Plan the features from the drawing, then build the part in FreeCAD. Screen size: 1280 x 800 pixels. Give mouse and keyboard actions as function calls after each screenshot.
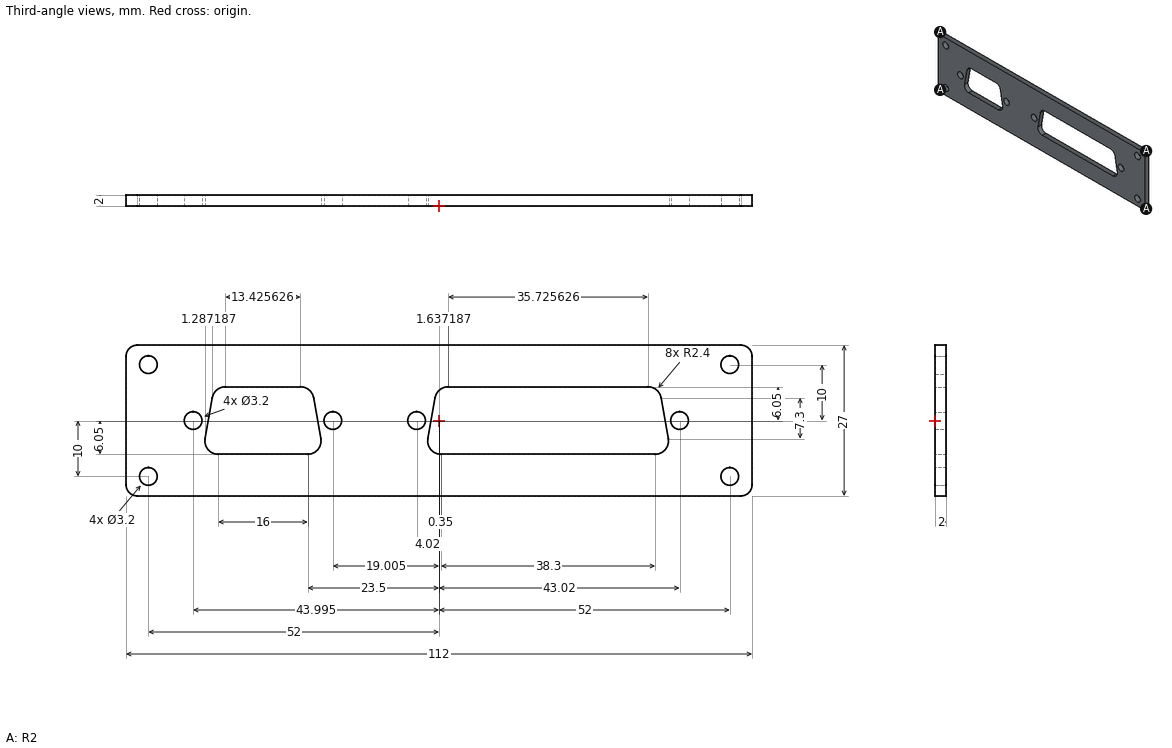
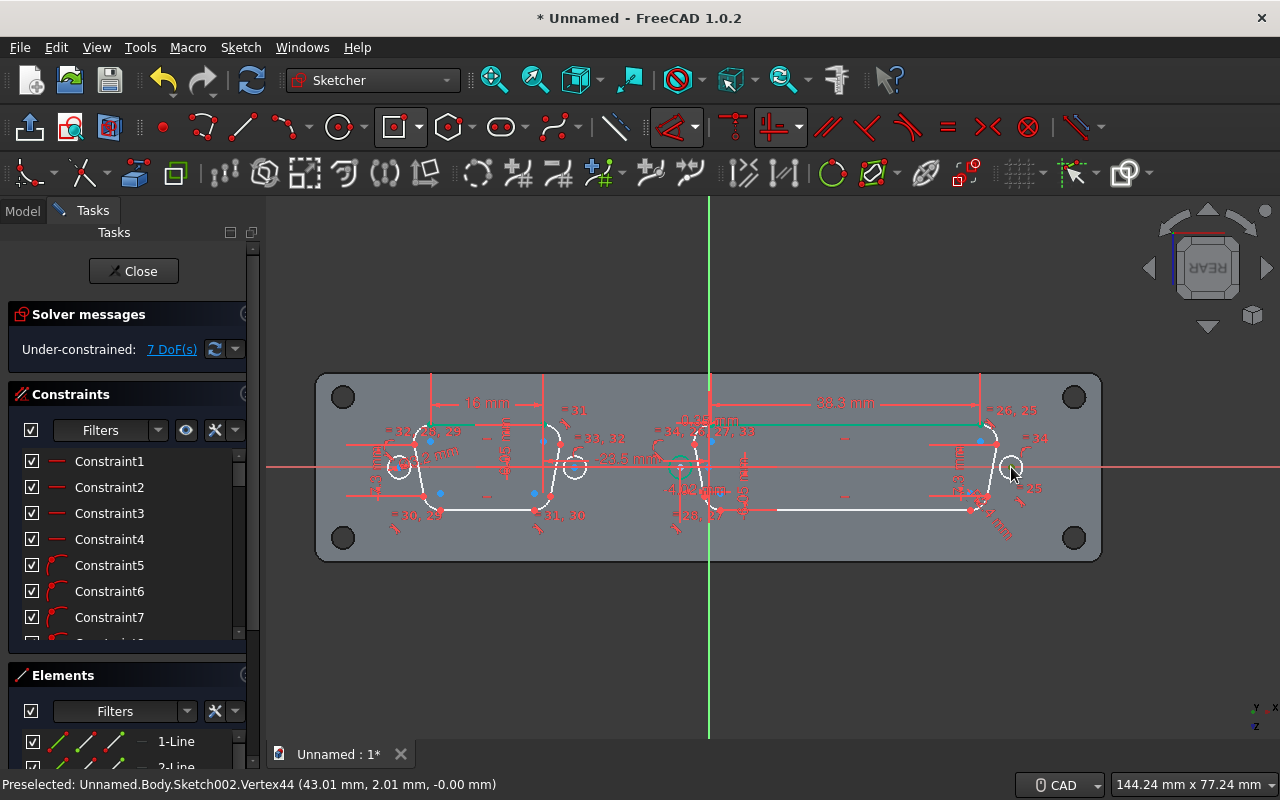
click(698, 128)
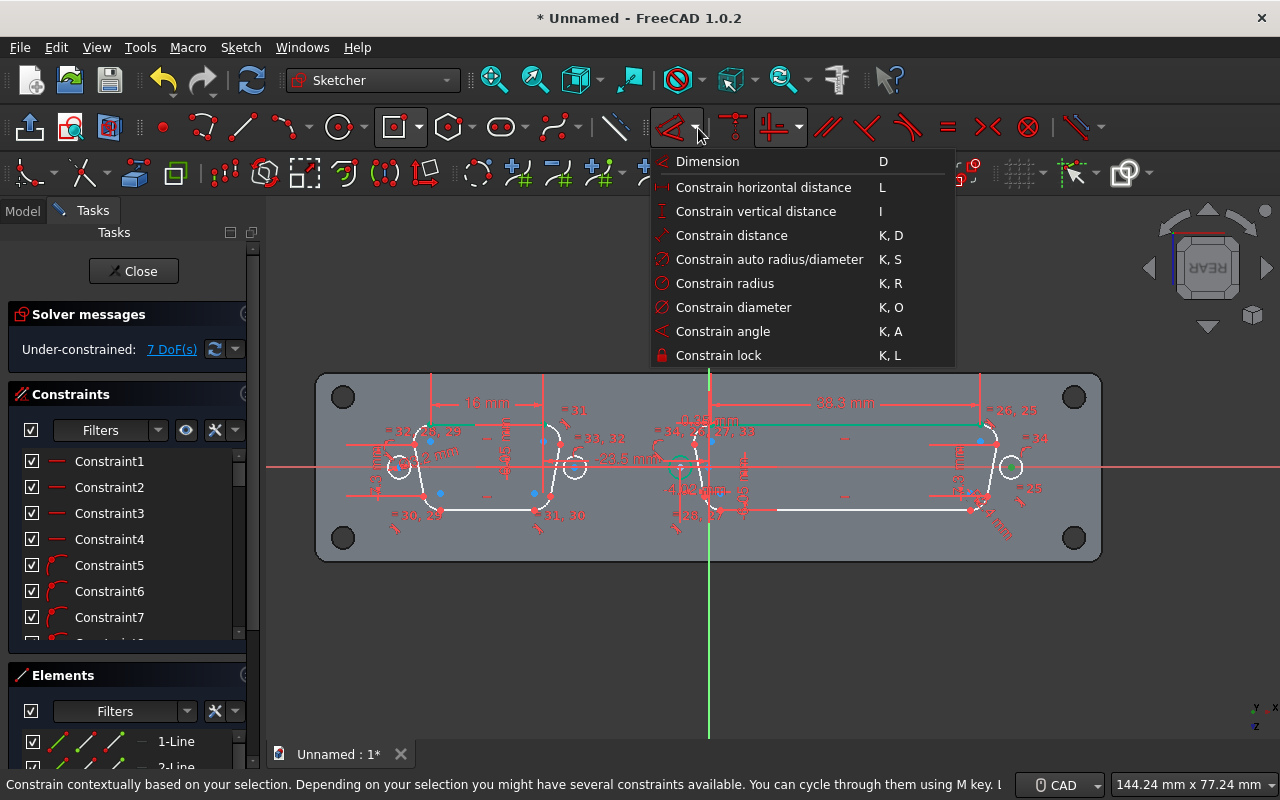
click(803, 187)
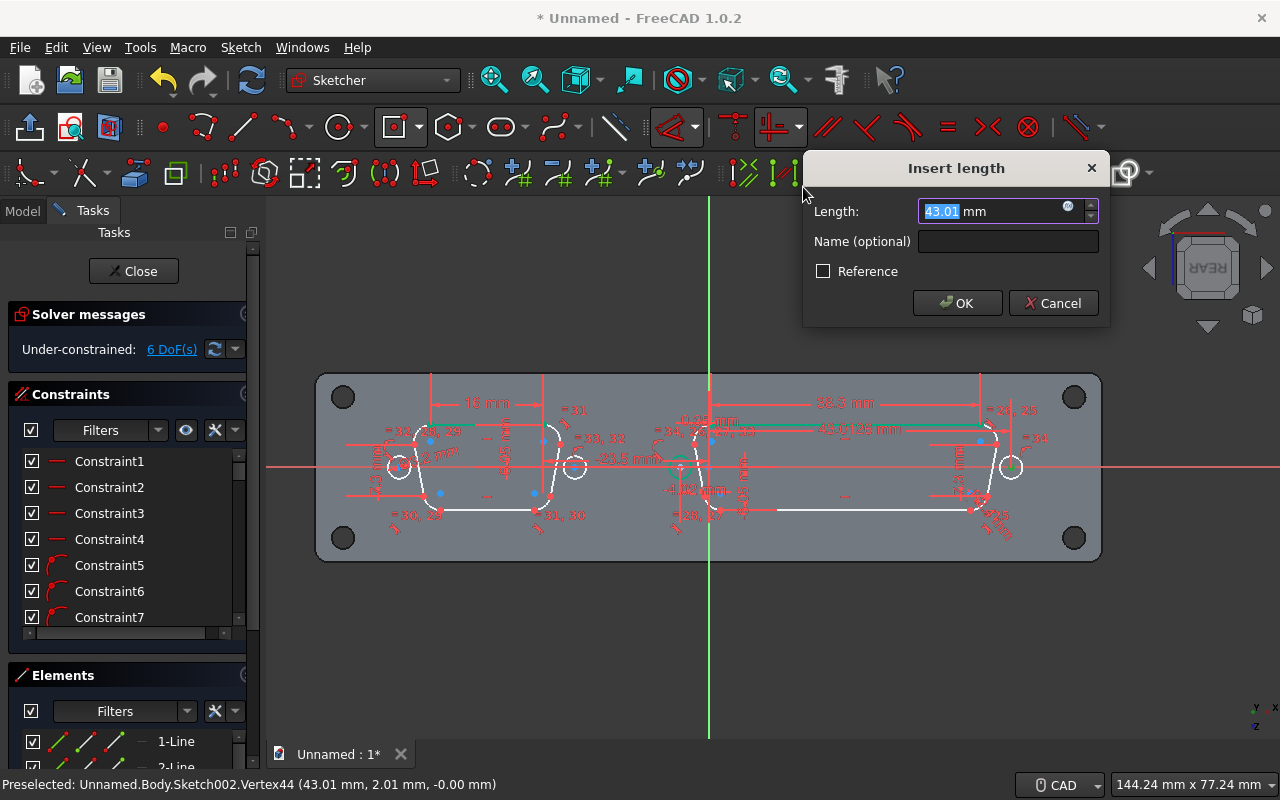
text(43.02)
key(Return)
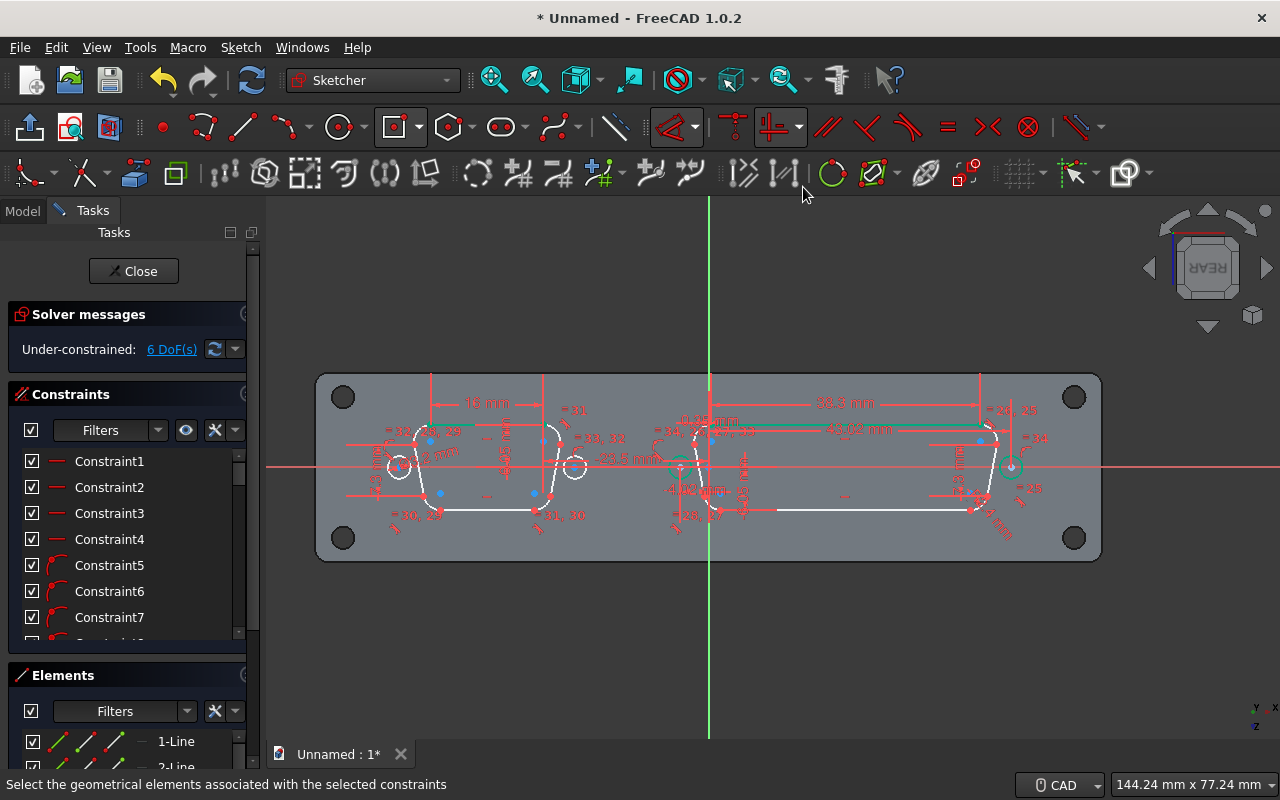
click(399, 467)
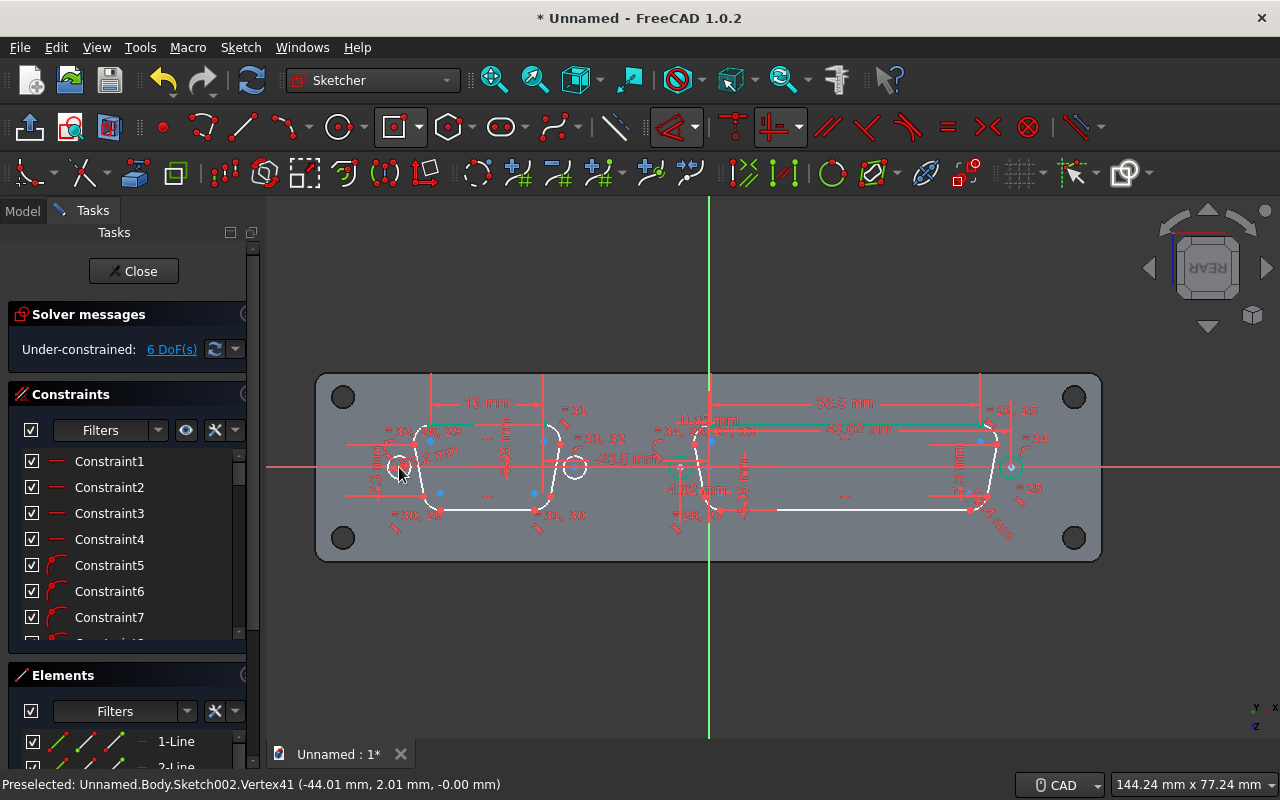
key(l)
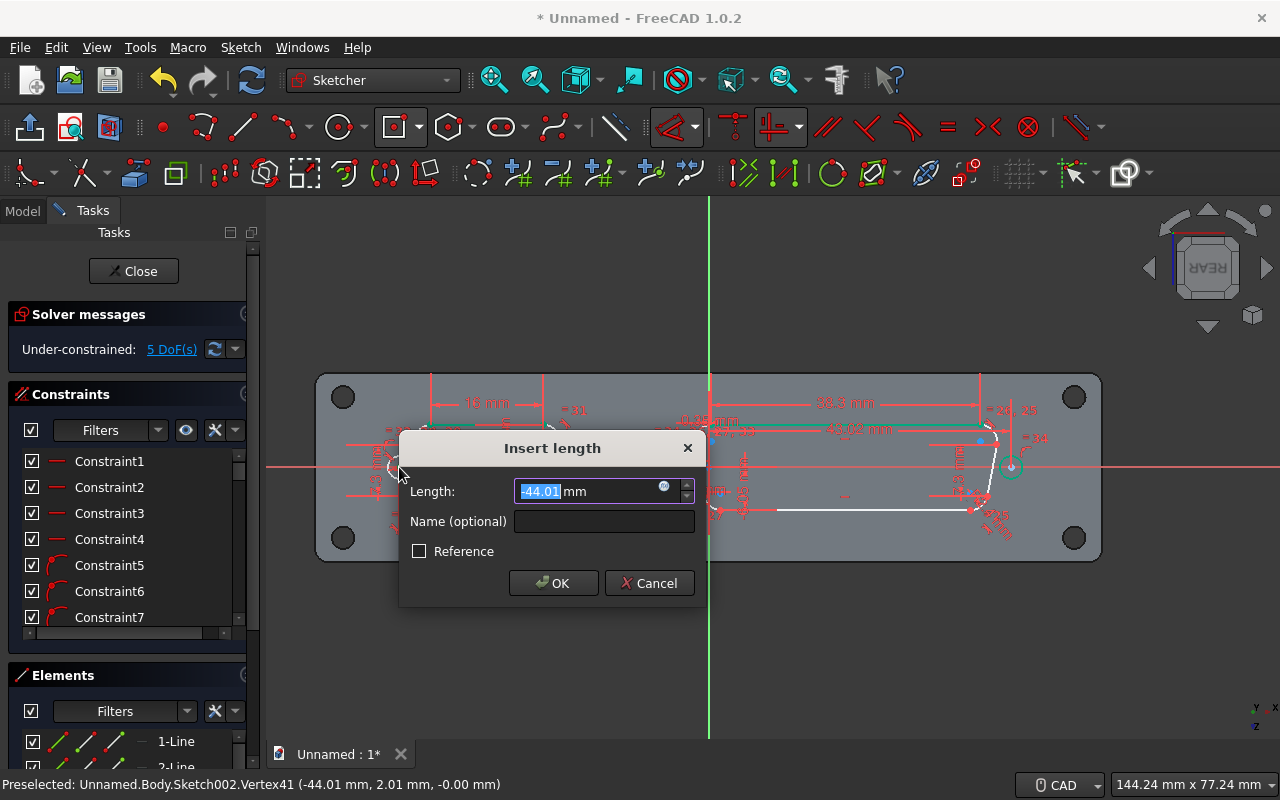
text(-43.995)
key(Return)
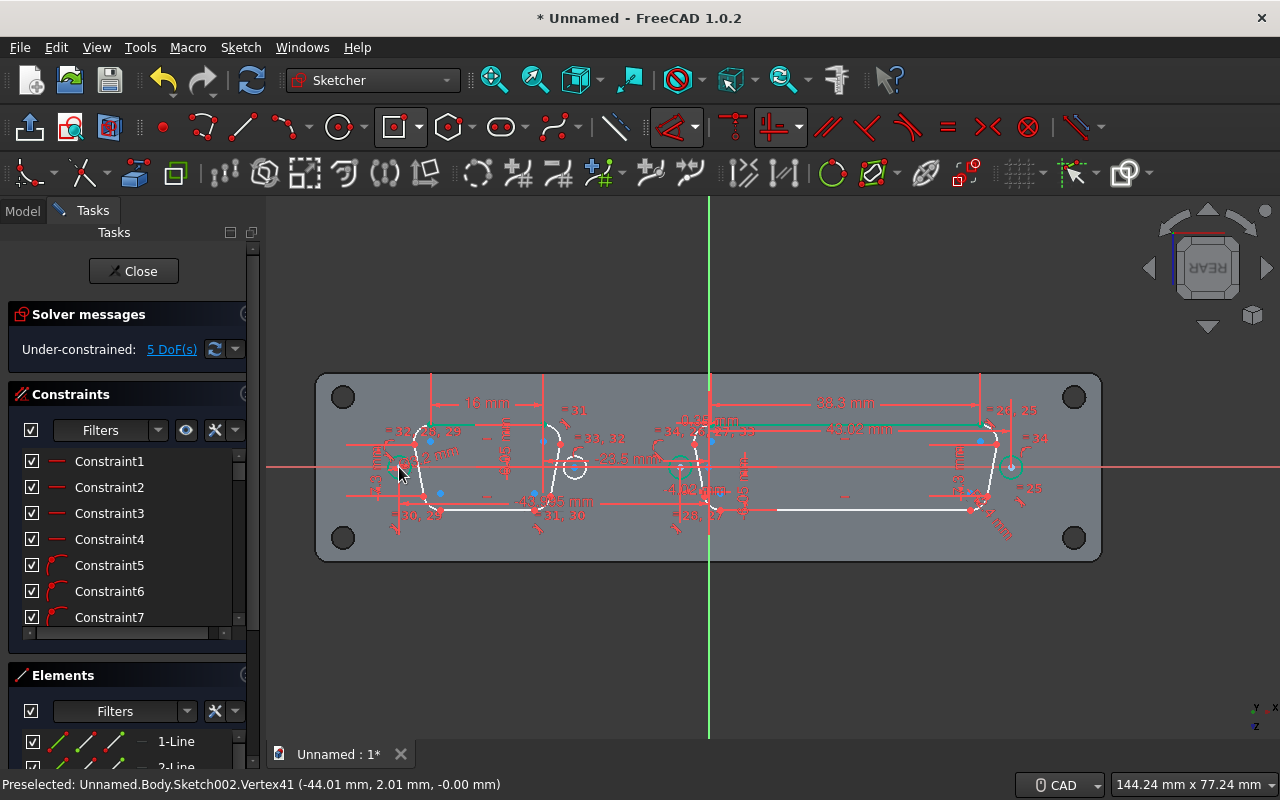
click(575, 467)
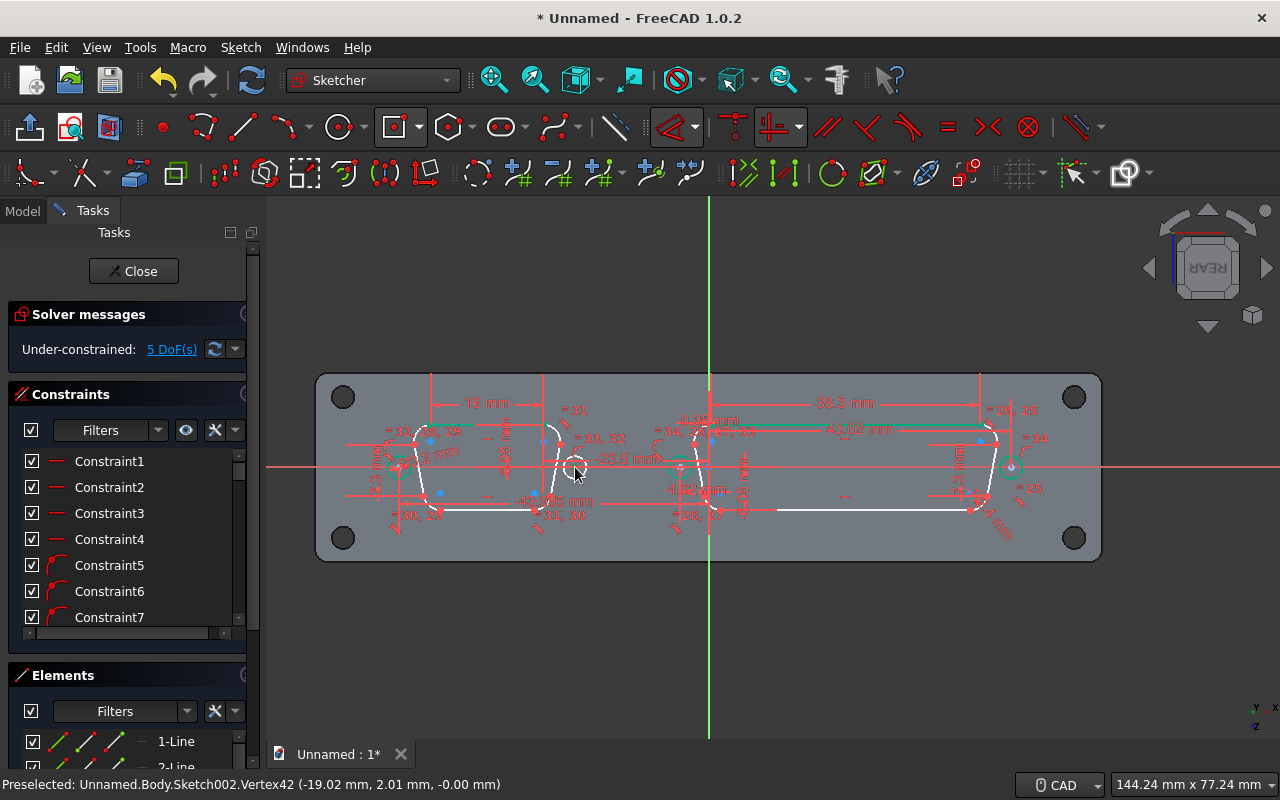
key(l)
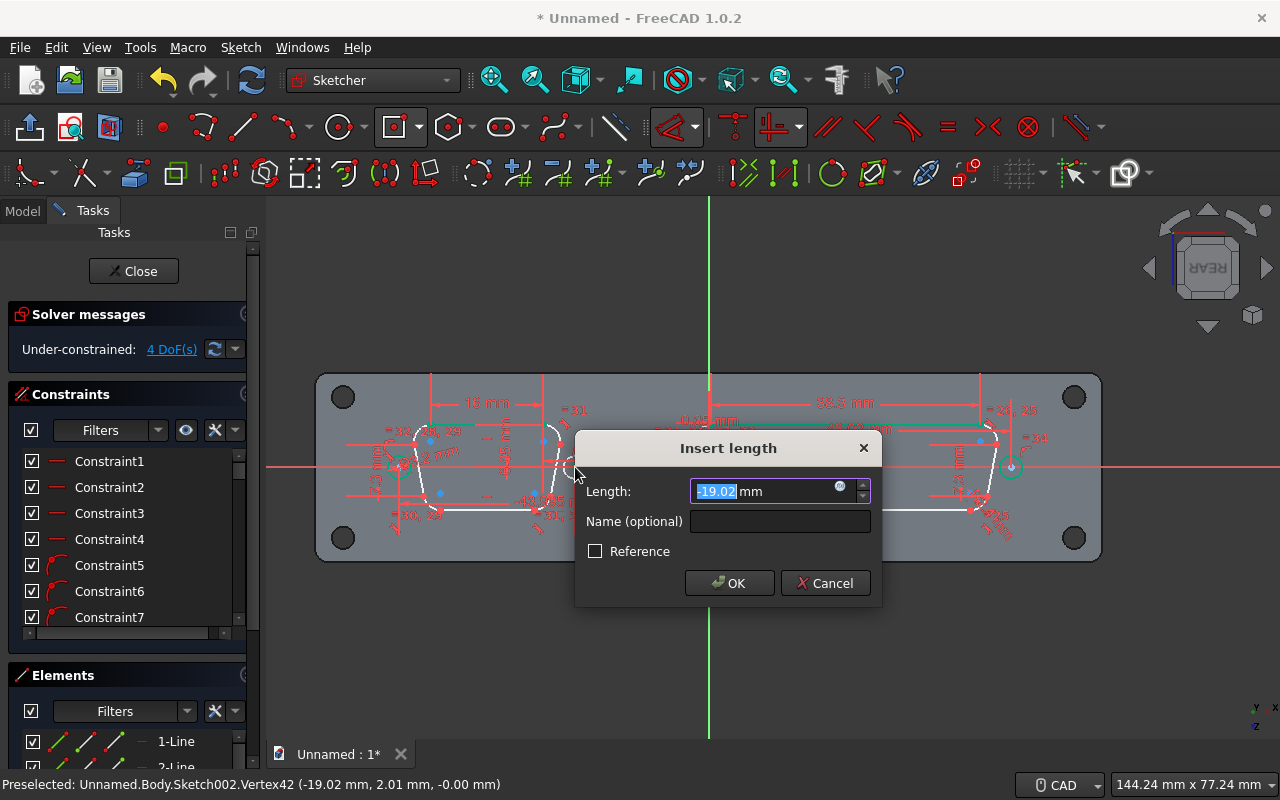
text(-19.005)
key(Return)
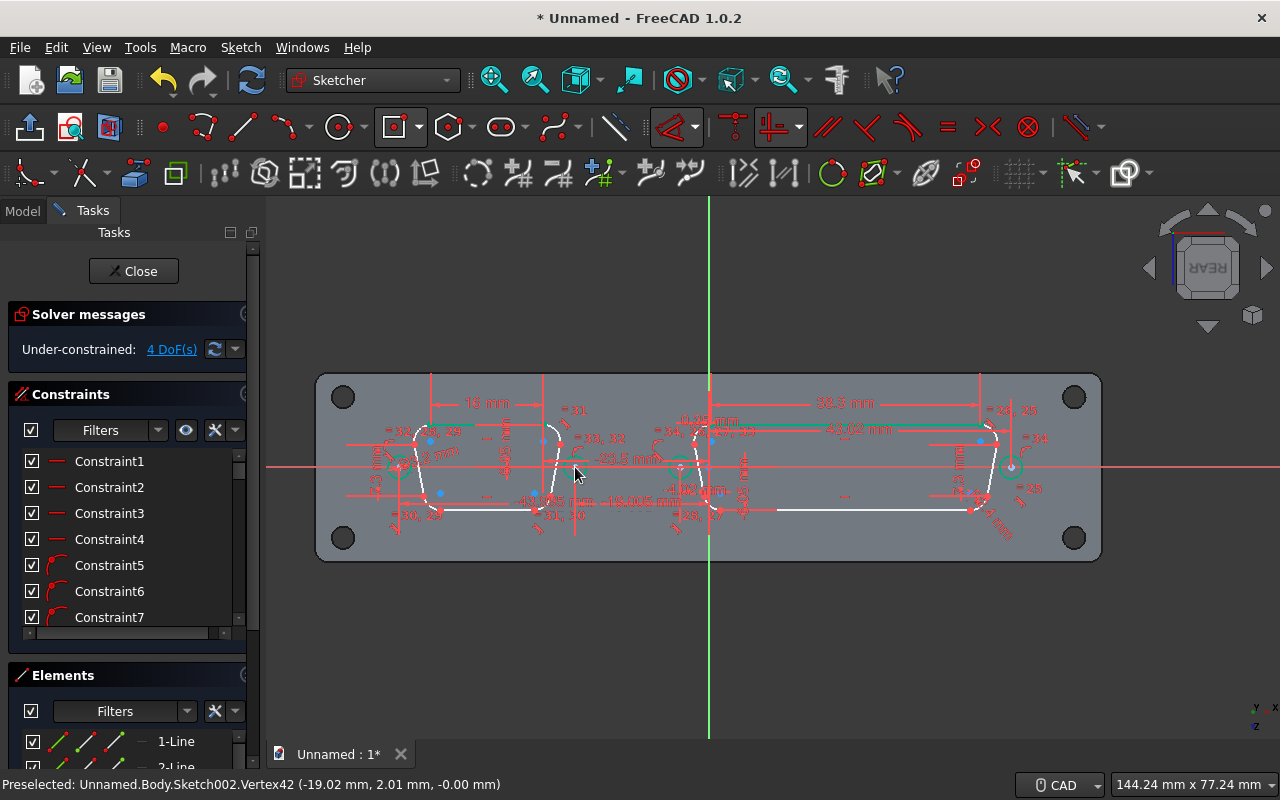
click(796, 510)